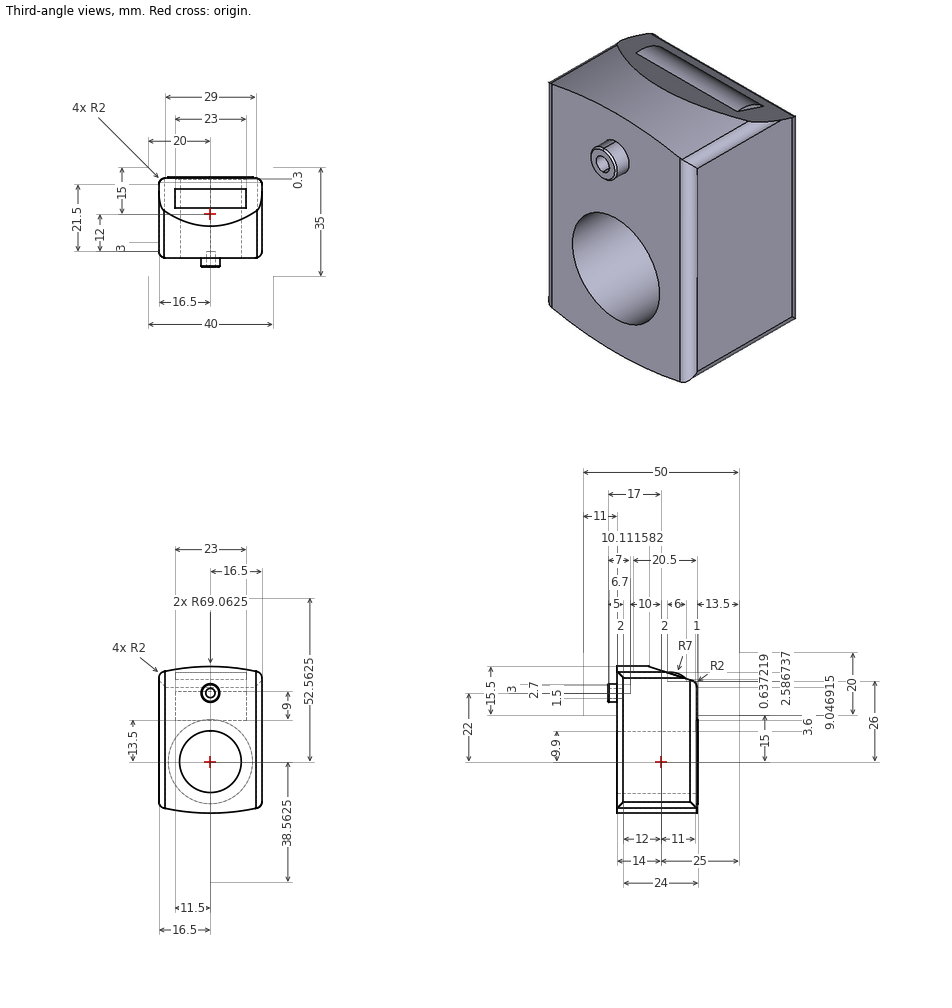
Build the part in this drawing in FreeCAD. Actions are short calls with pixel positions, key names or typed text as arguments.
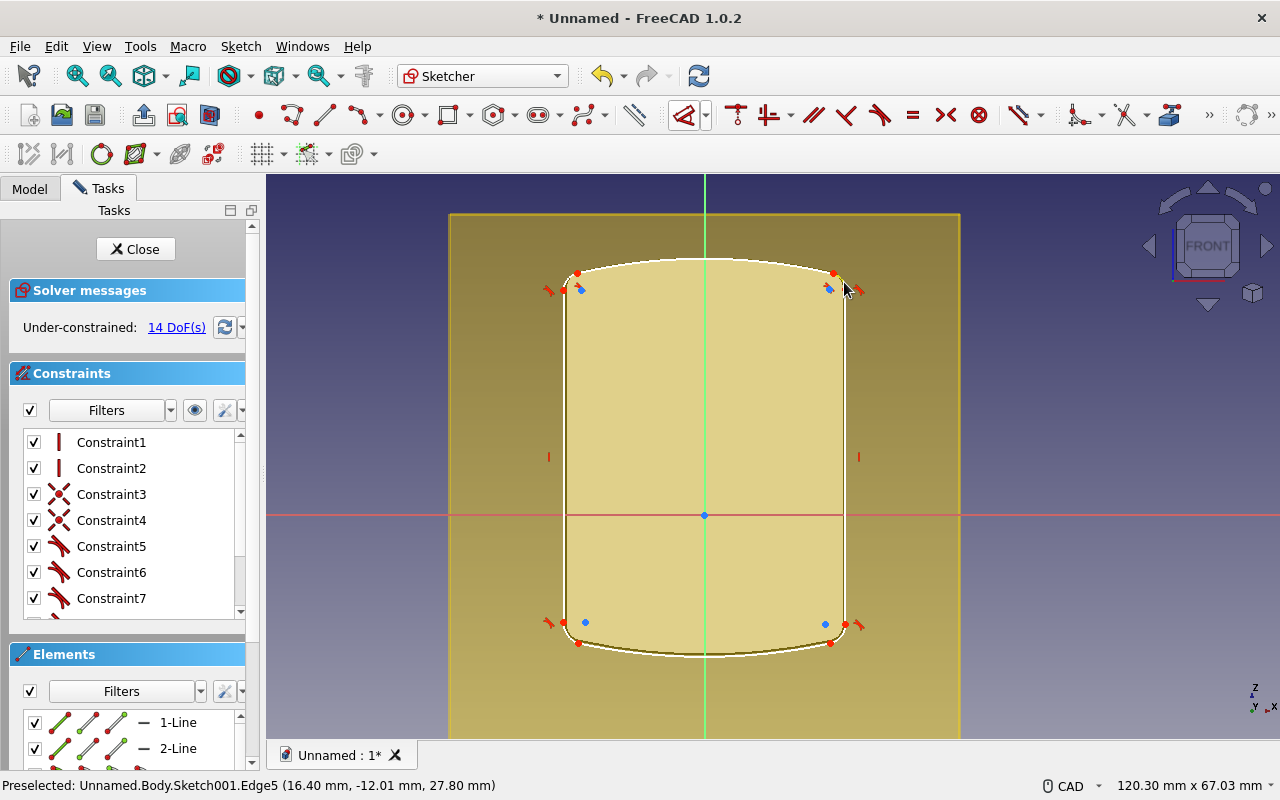
scroll(838, 640, up, 3)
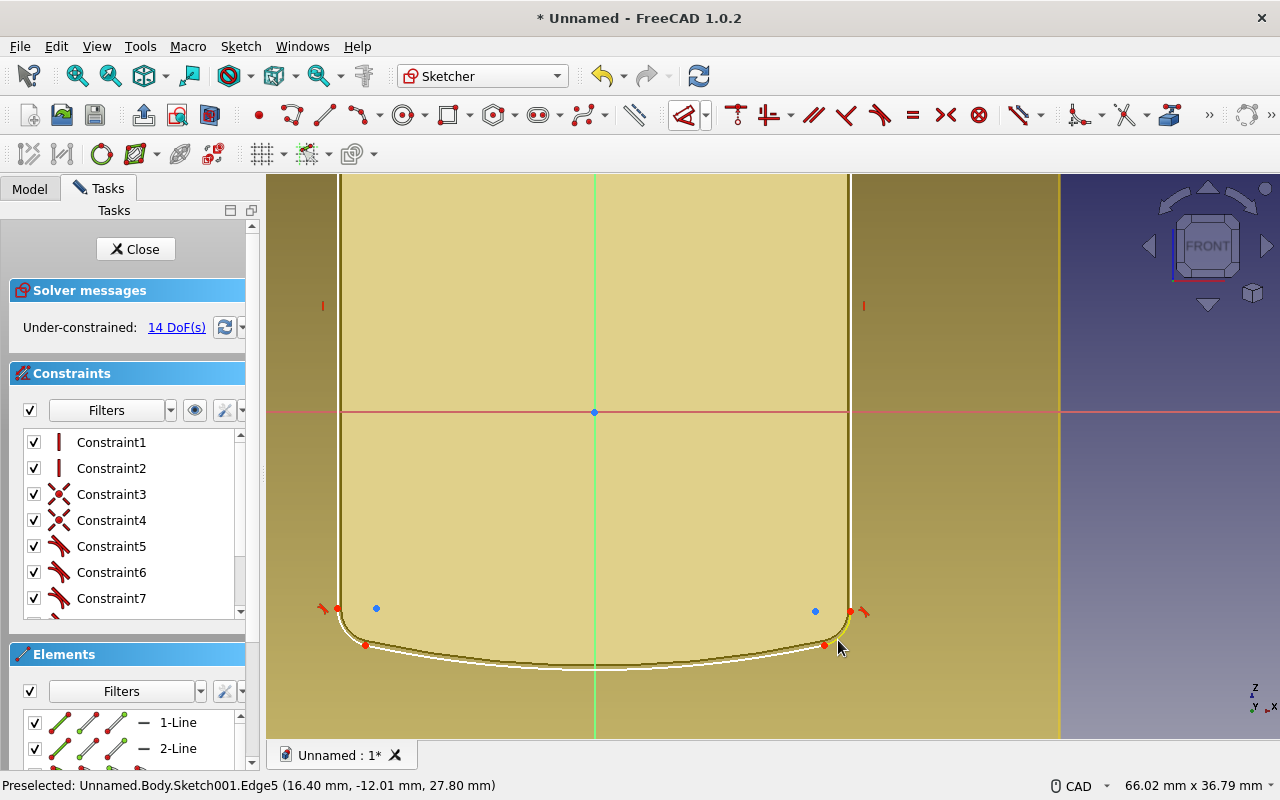
click(837, 639)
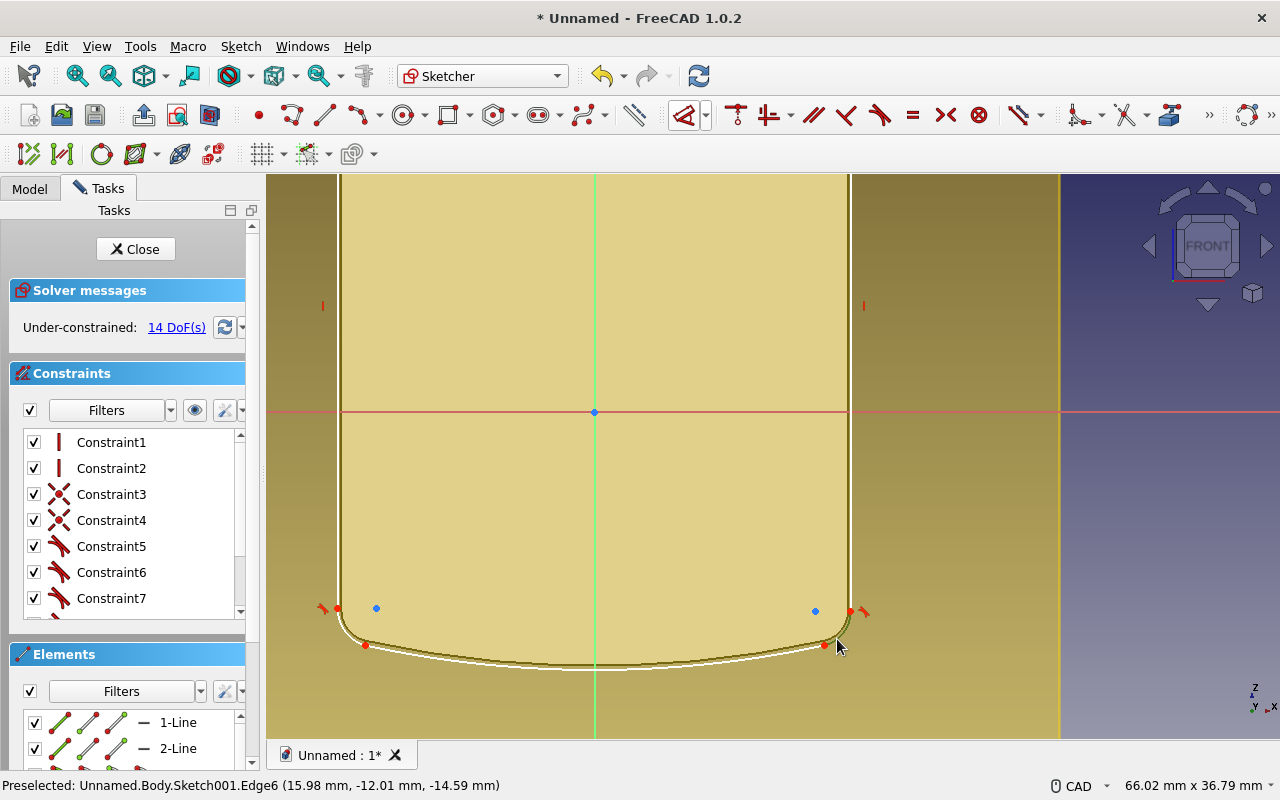
click(502, 666)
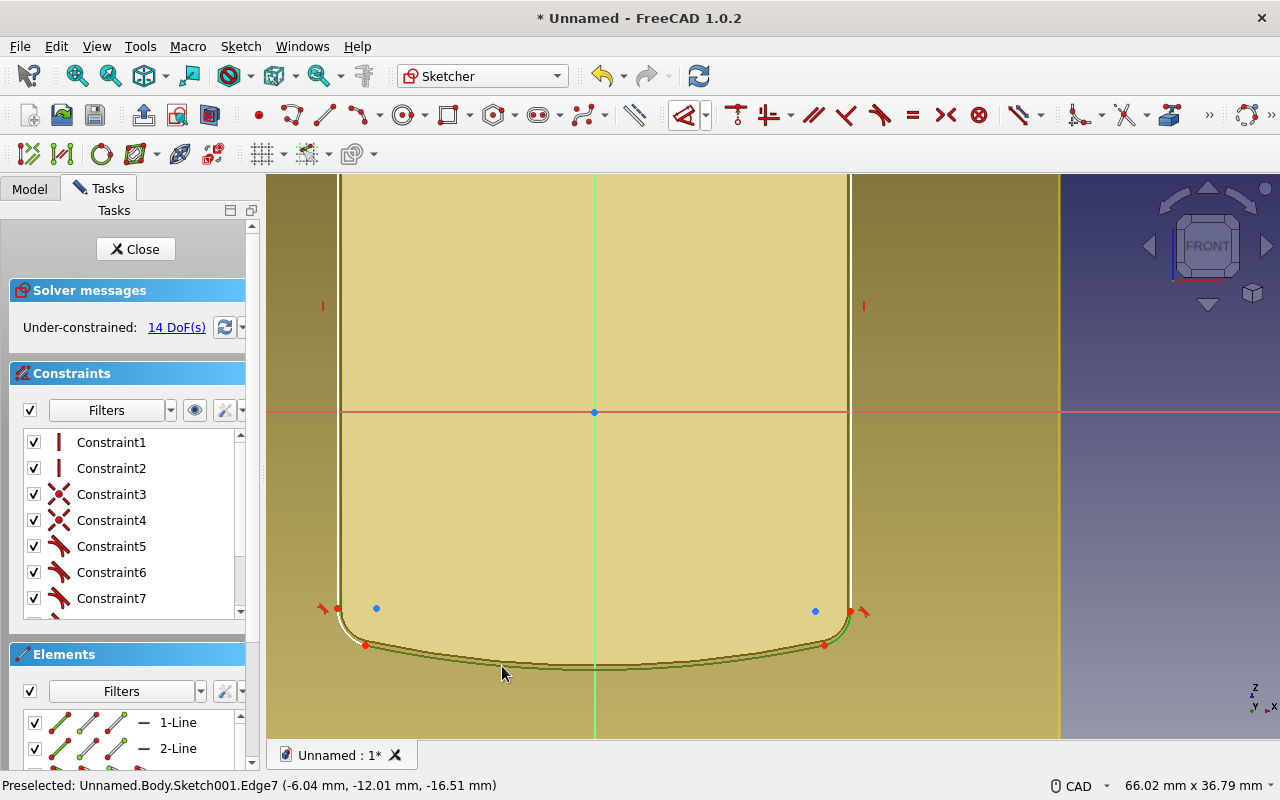
click(880, 116)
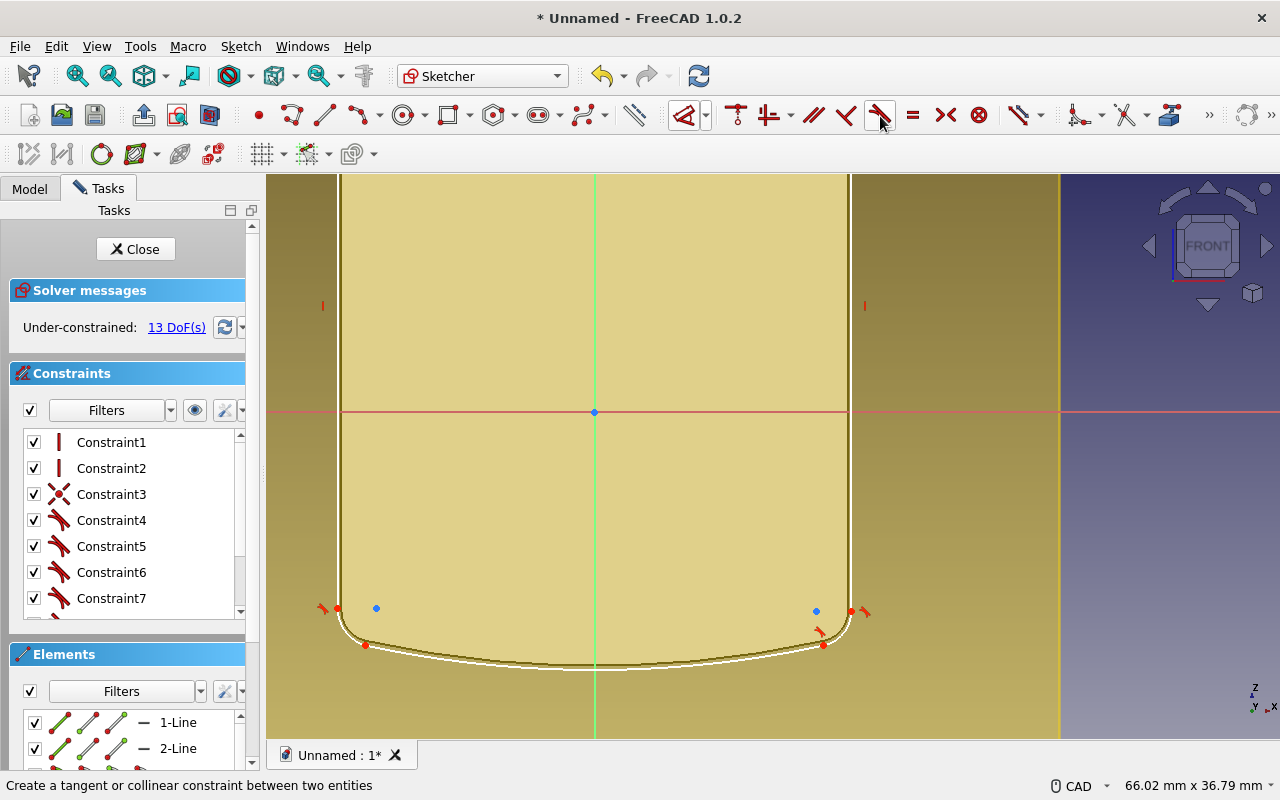
click(502, 666)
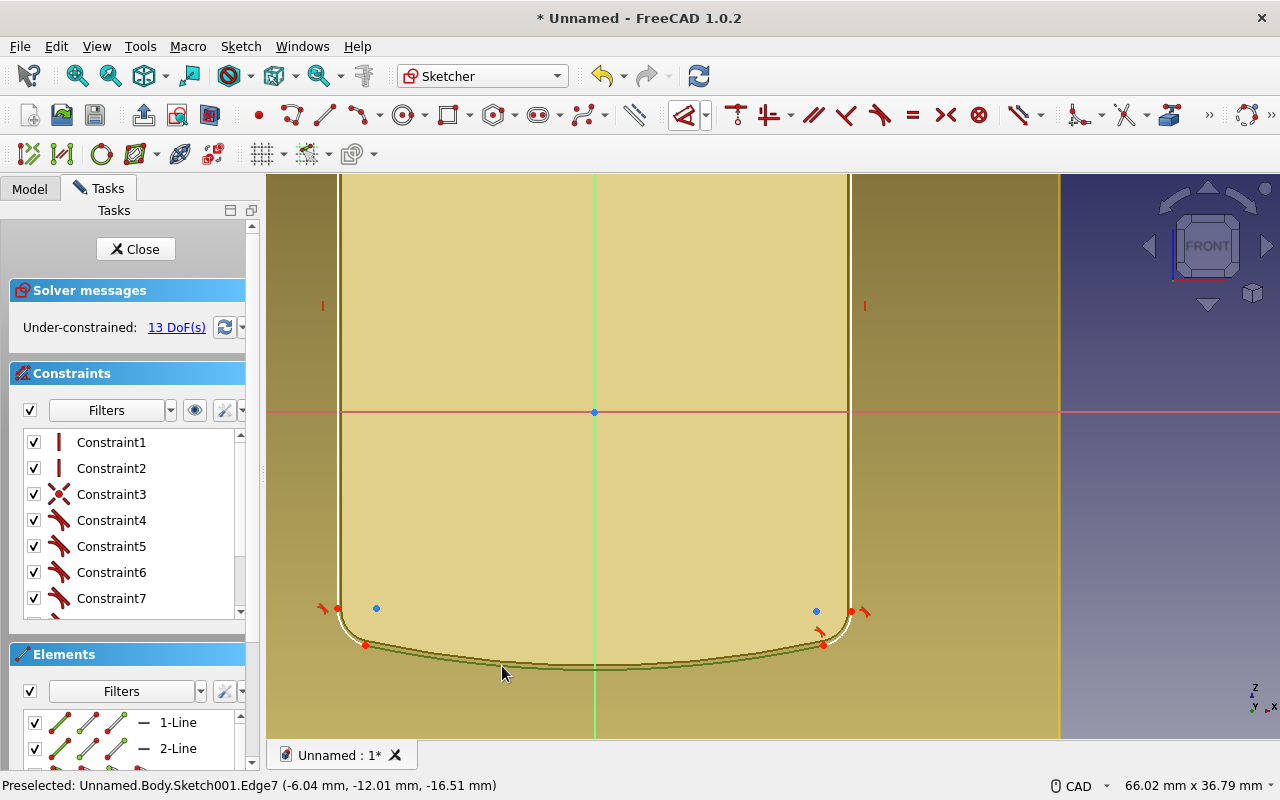
click(341, 623)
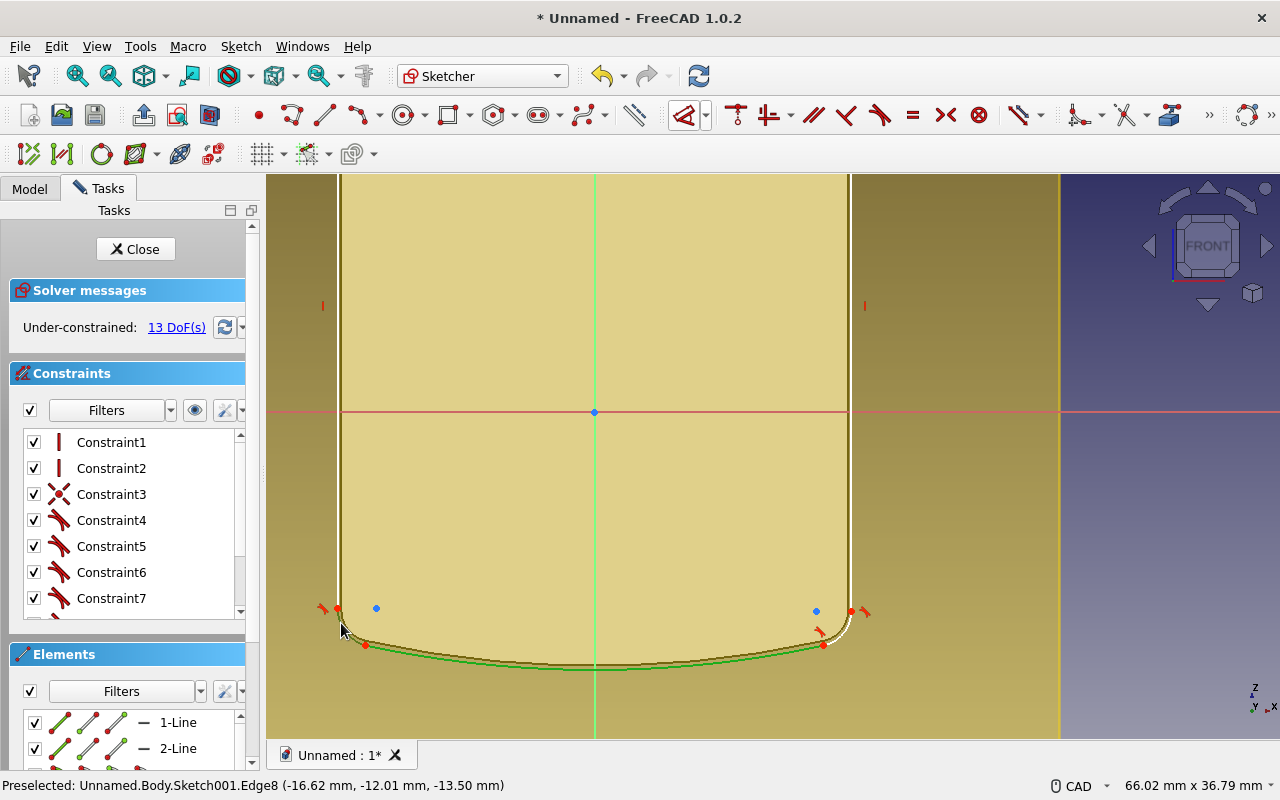
click(880, 116)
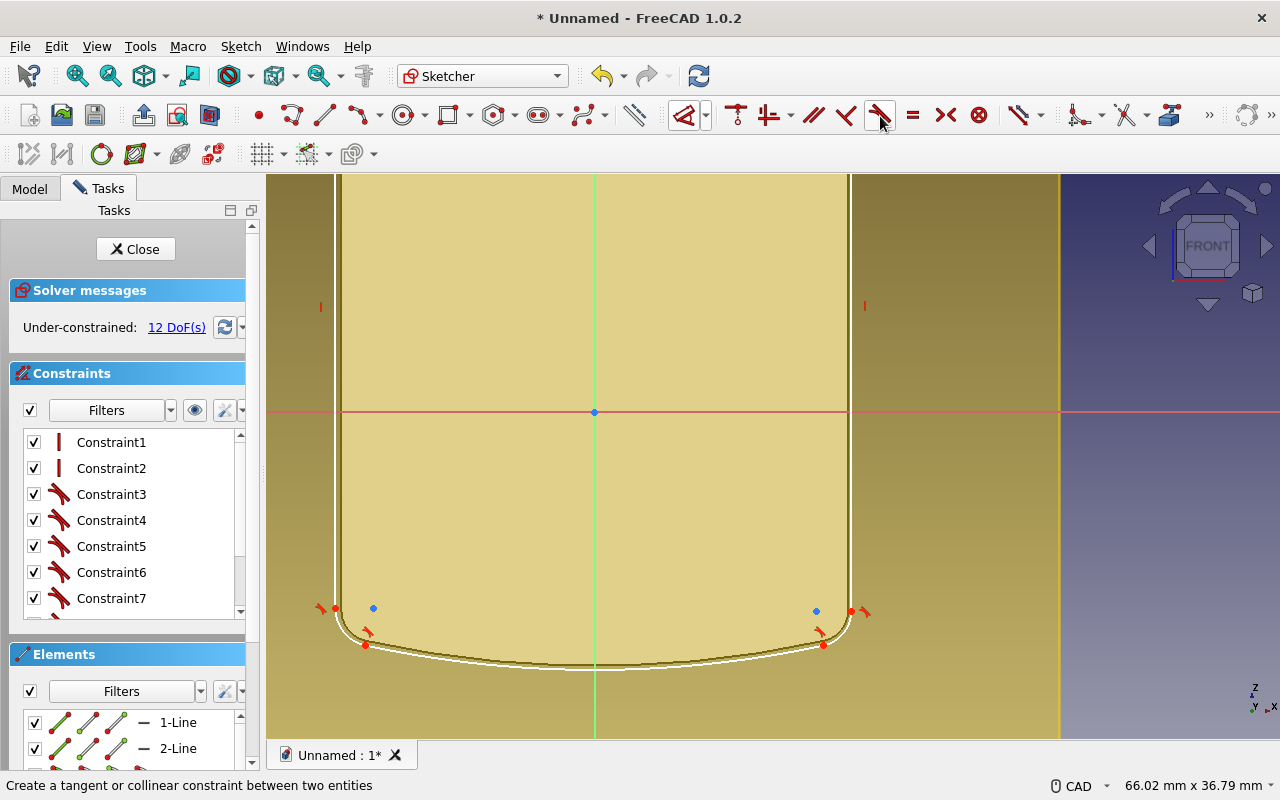
scroll(838, 641, down, 3)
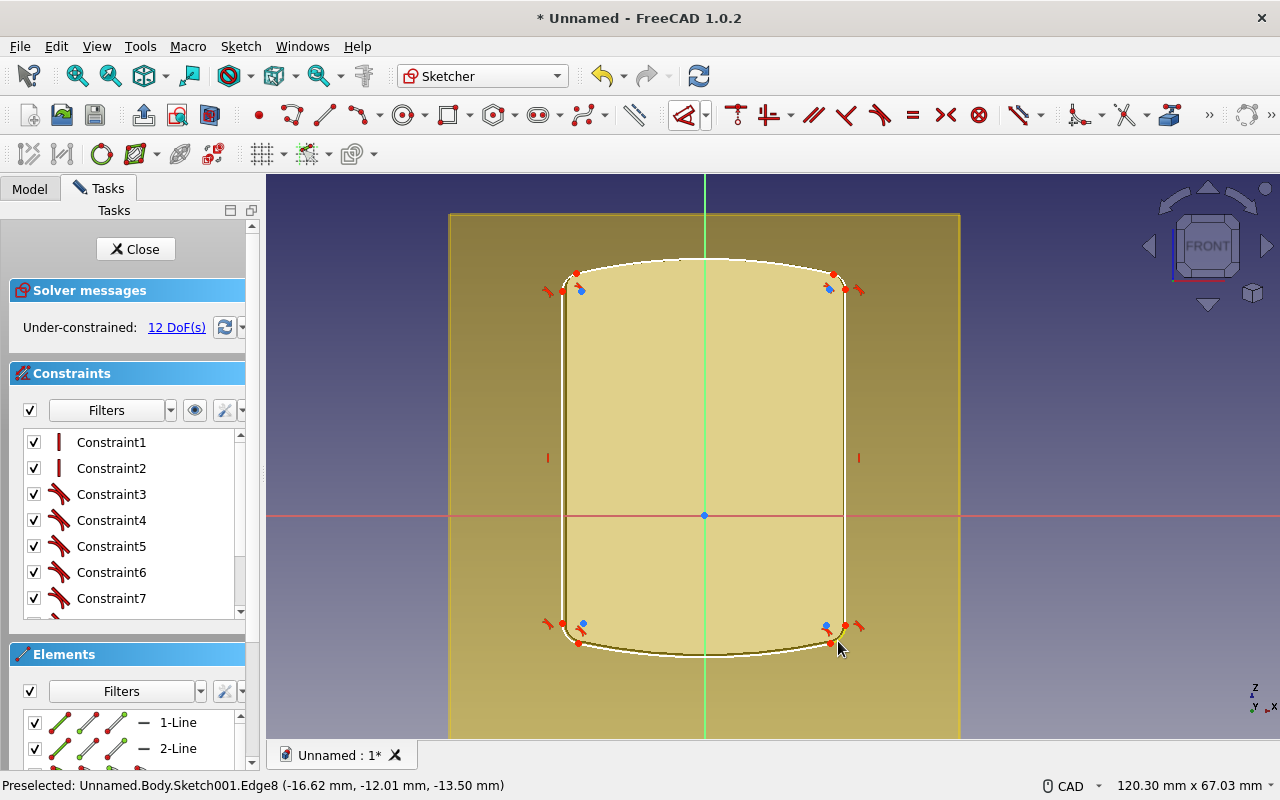
scroll(570, 277, up, 4)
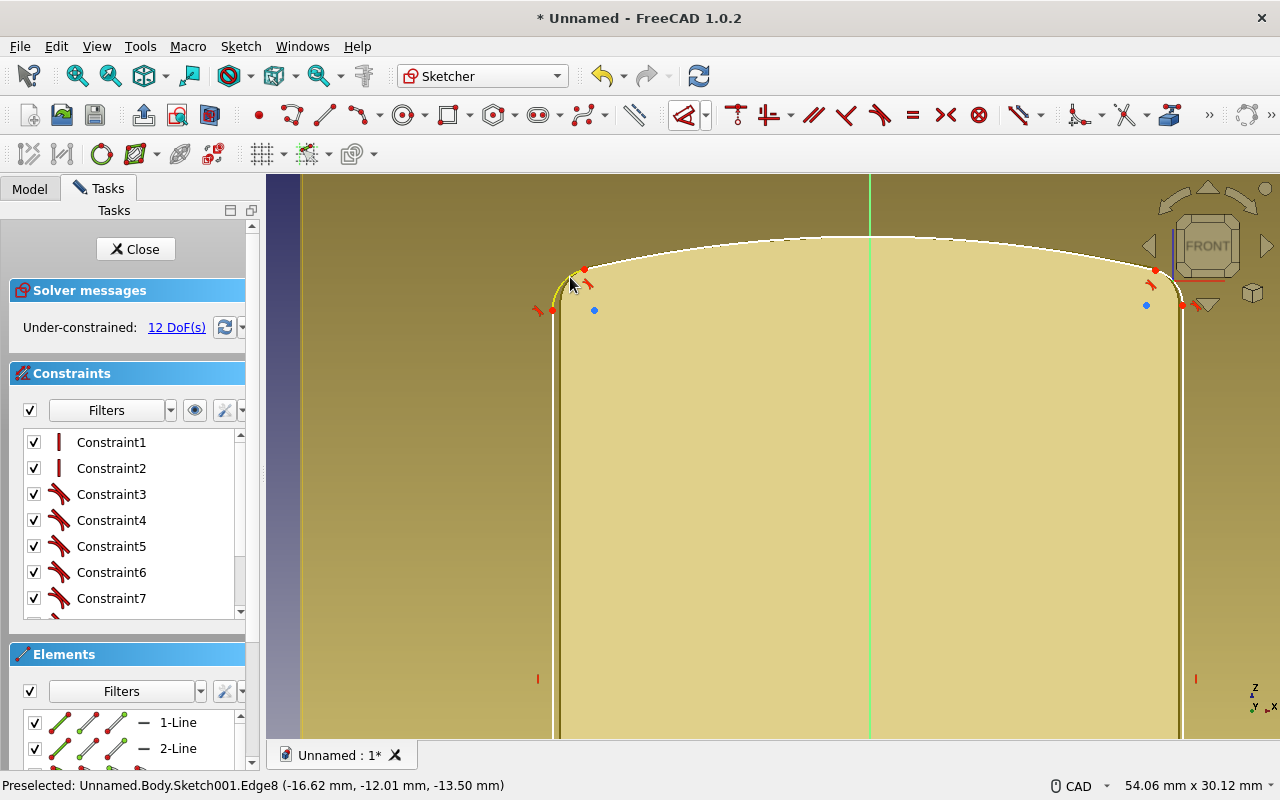
click(570, 276)